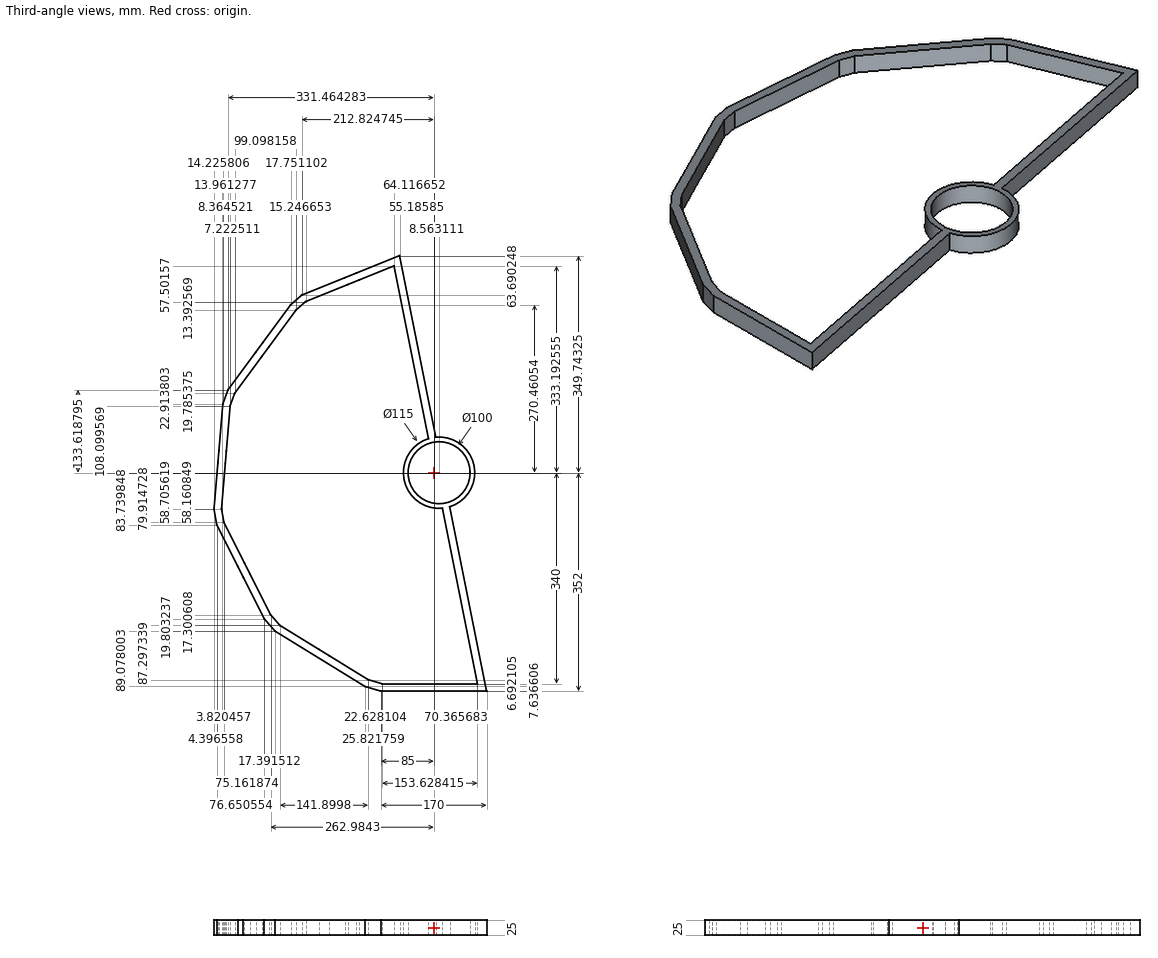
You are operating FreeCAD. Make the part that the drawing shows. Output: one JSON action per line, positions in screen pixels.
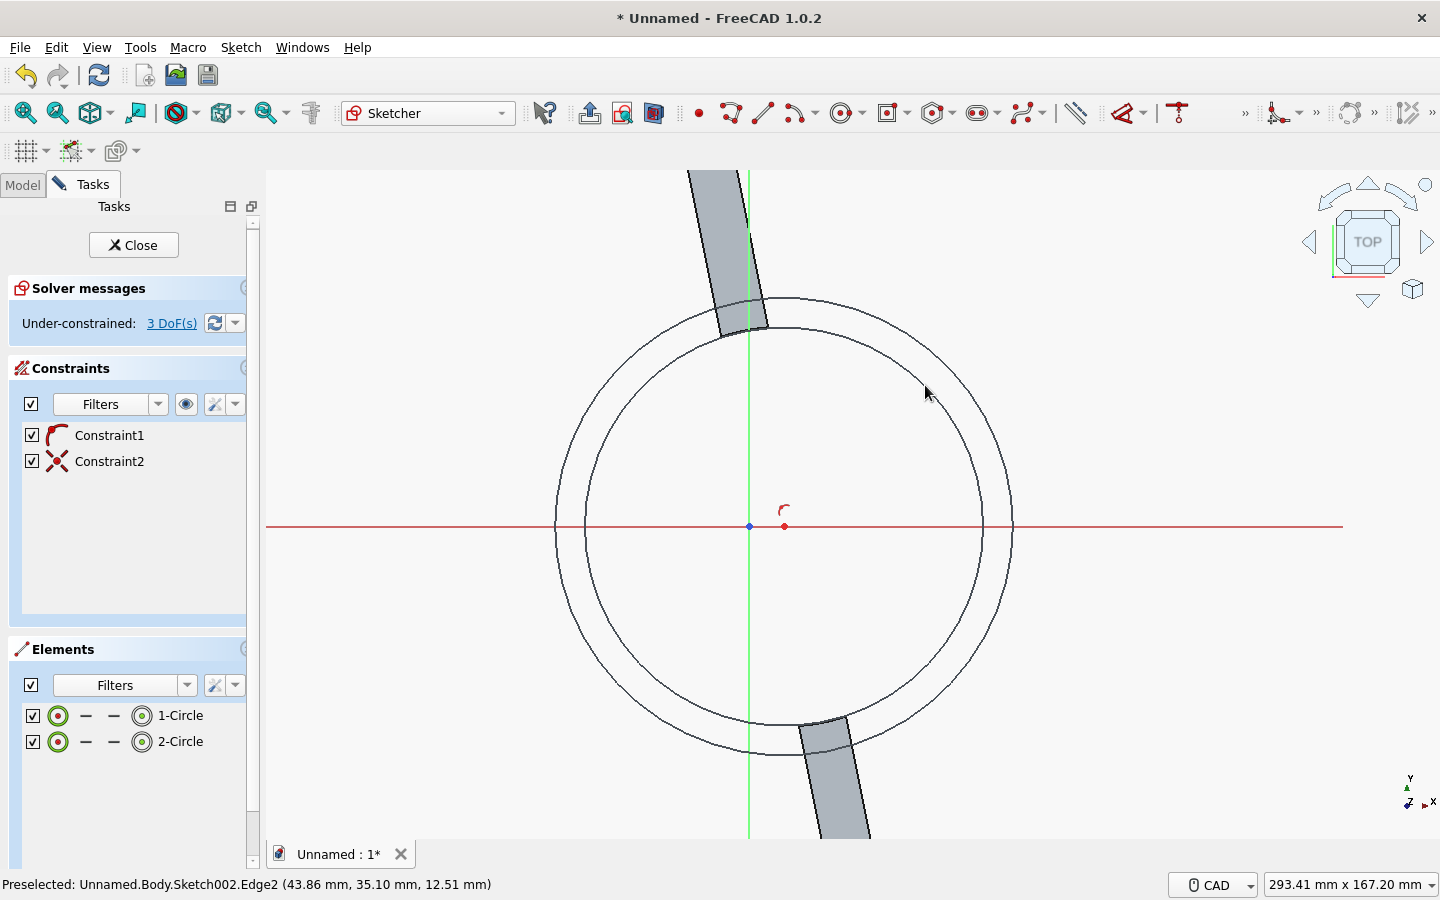
{"action": "left_click", "coordinate": [1122, 114]}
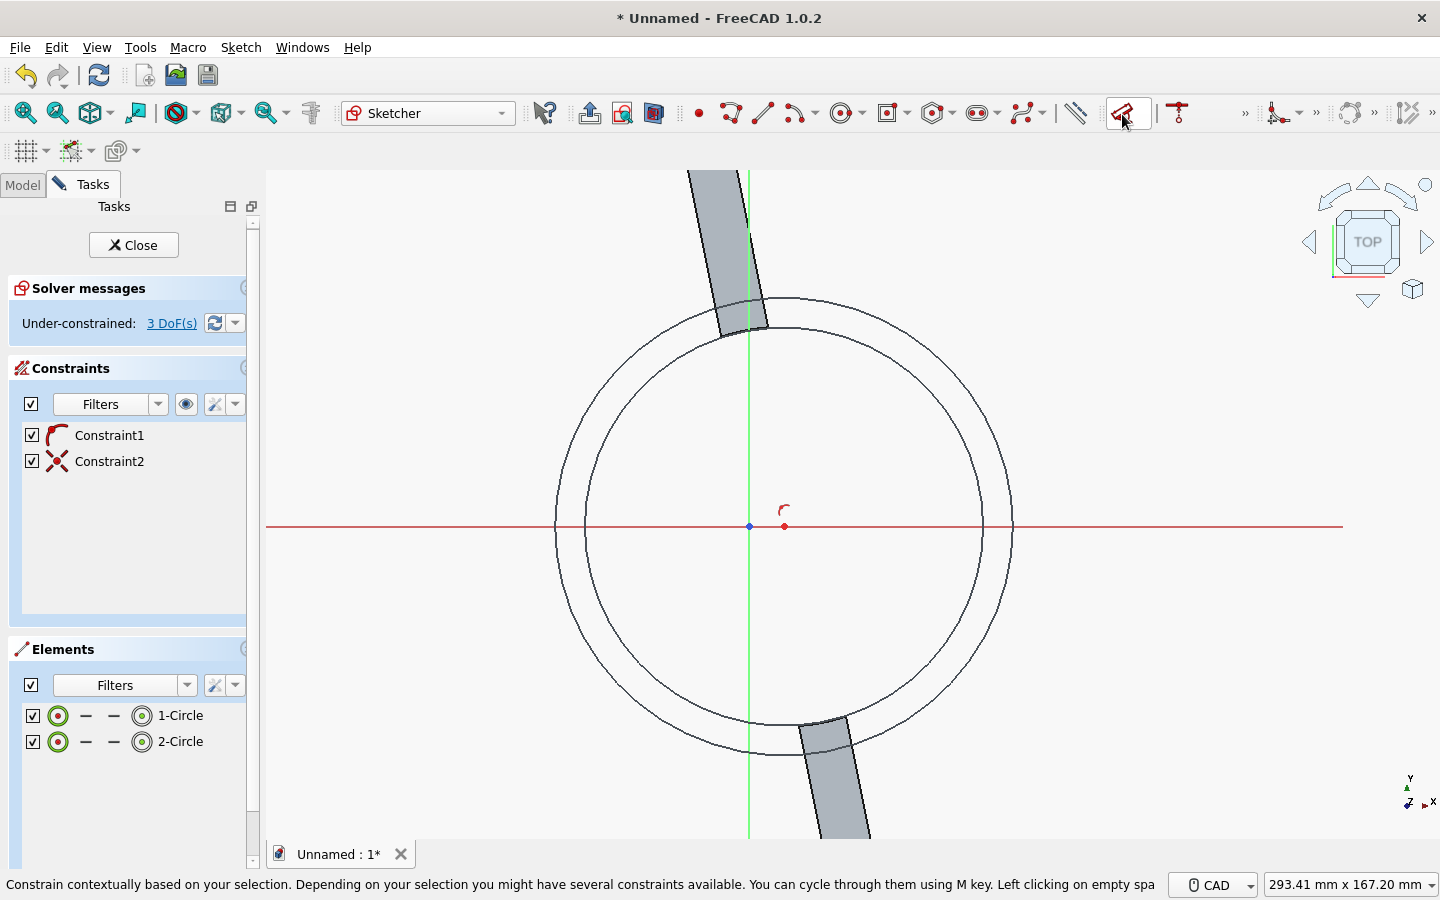
{"action": "left_click", "coordinate": [945, 364]}
{"action": "left_click", "coordinate": [968, 341]}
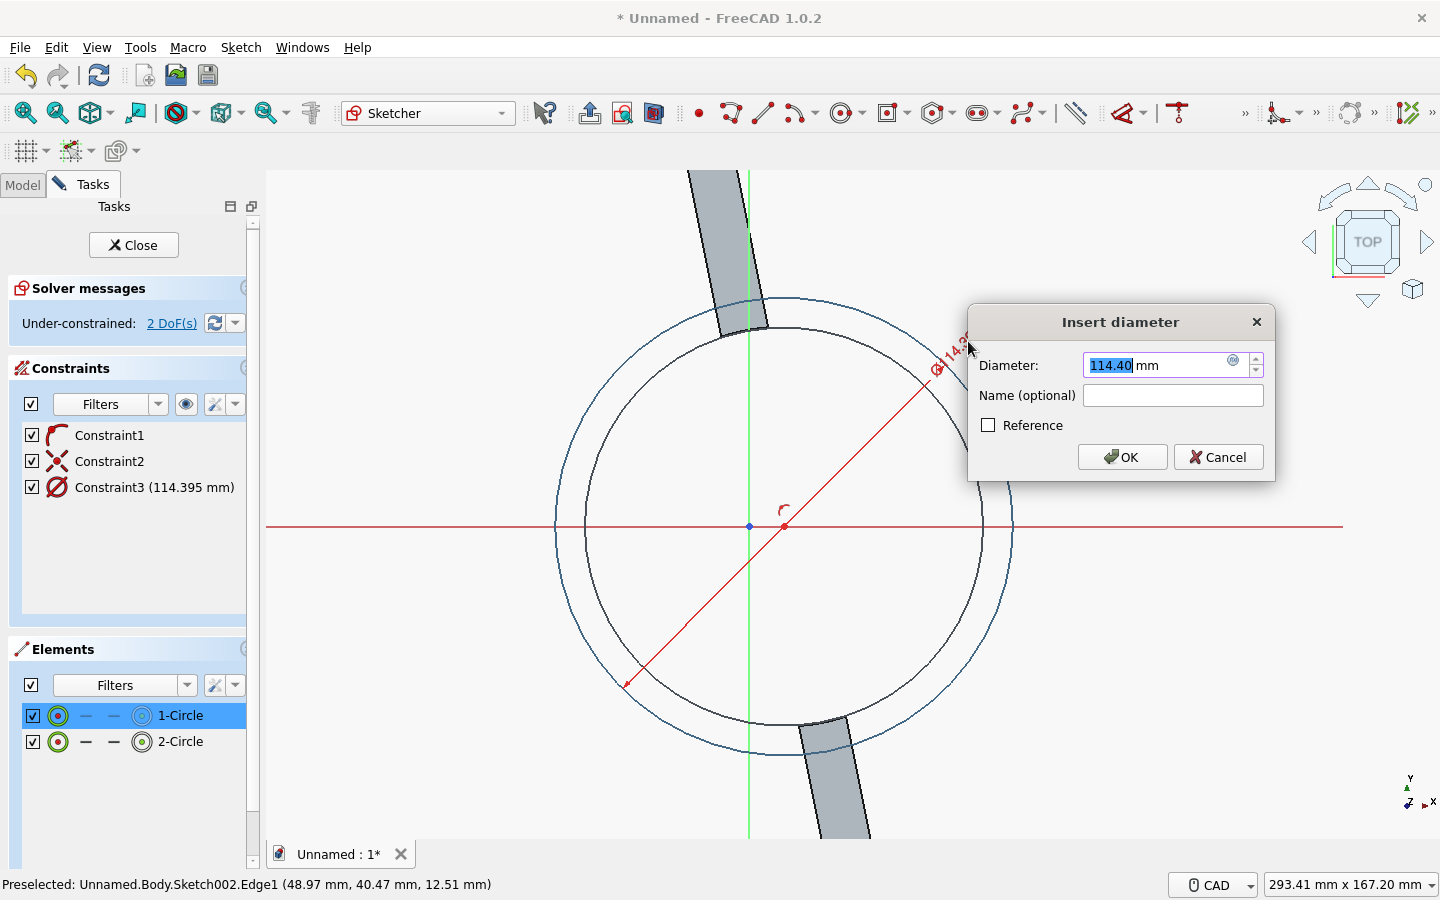
{"action": "type", "text": "115"}
{"action": "key", "text": "Return"}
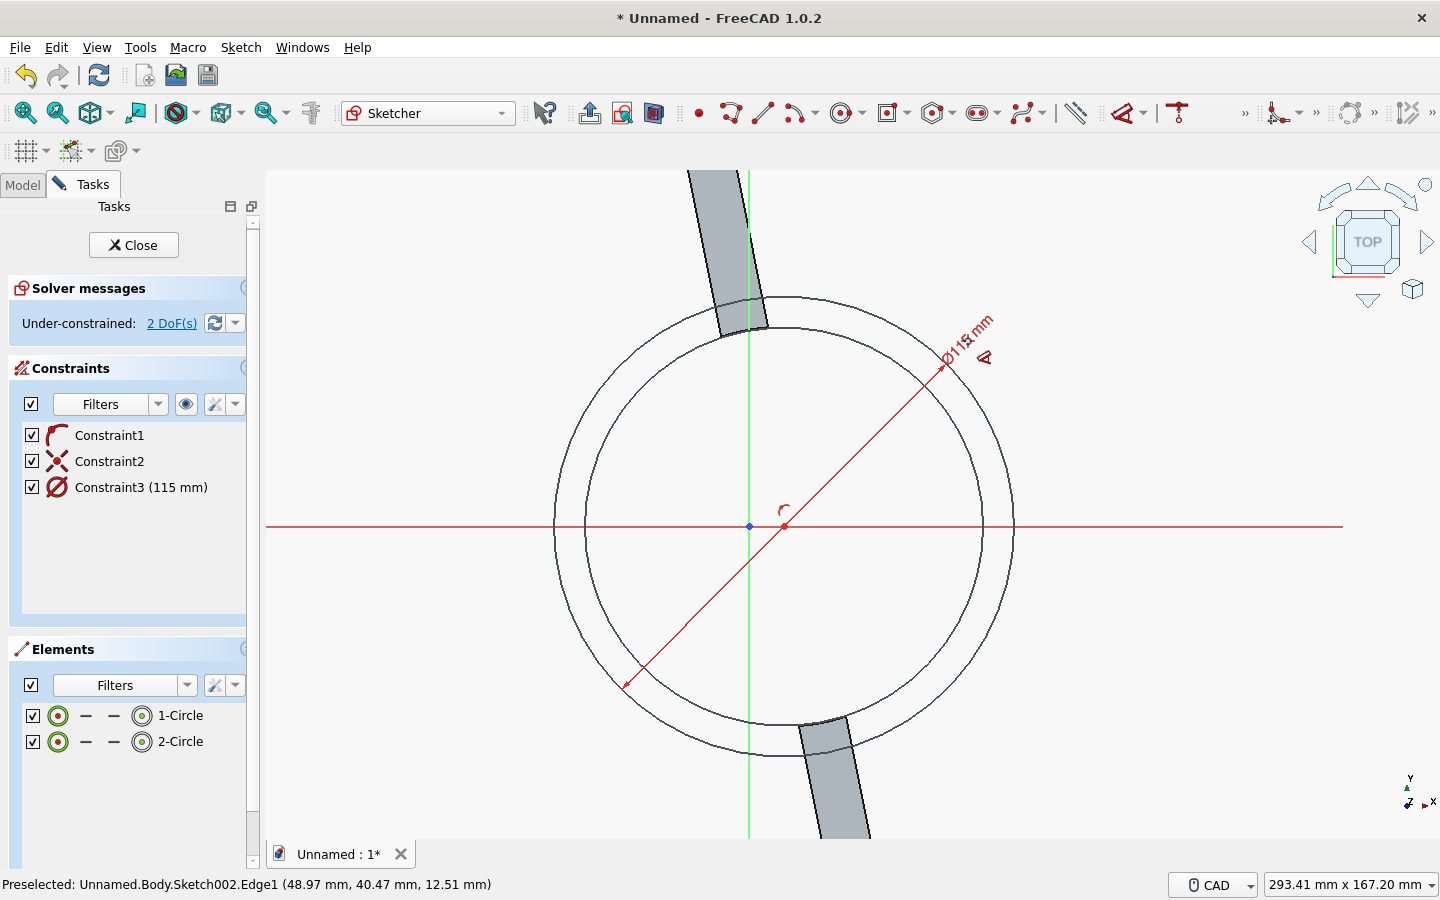
{"action": "left_click", "coordinate": [924, 385]}
{"action": "left_click", "coordinate": [1027, 454]}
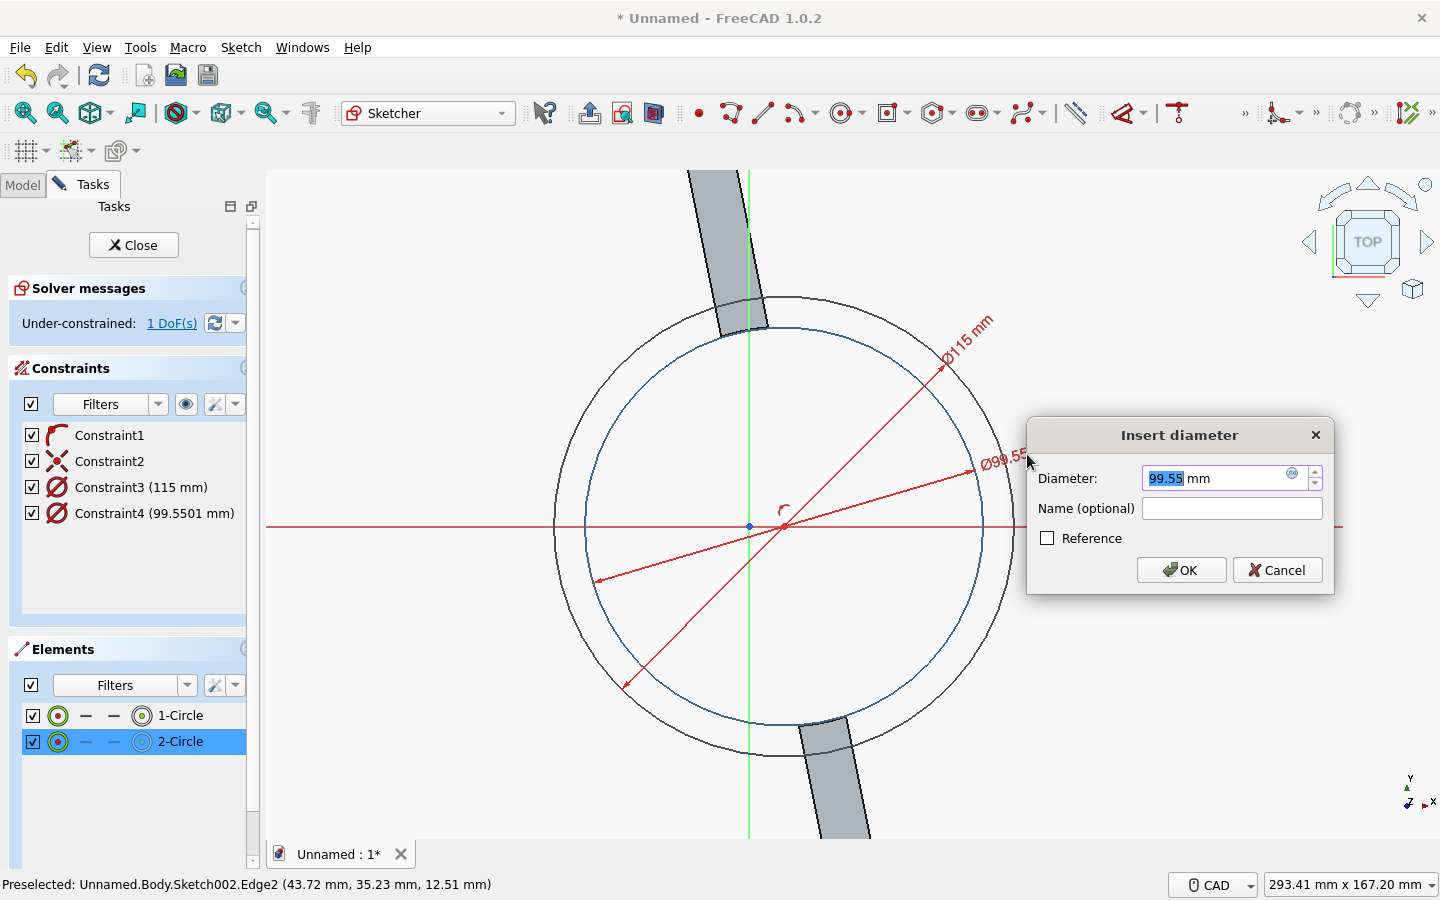
{"action": "type", "text": "100"}
{"action": "key", "text": "Return"}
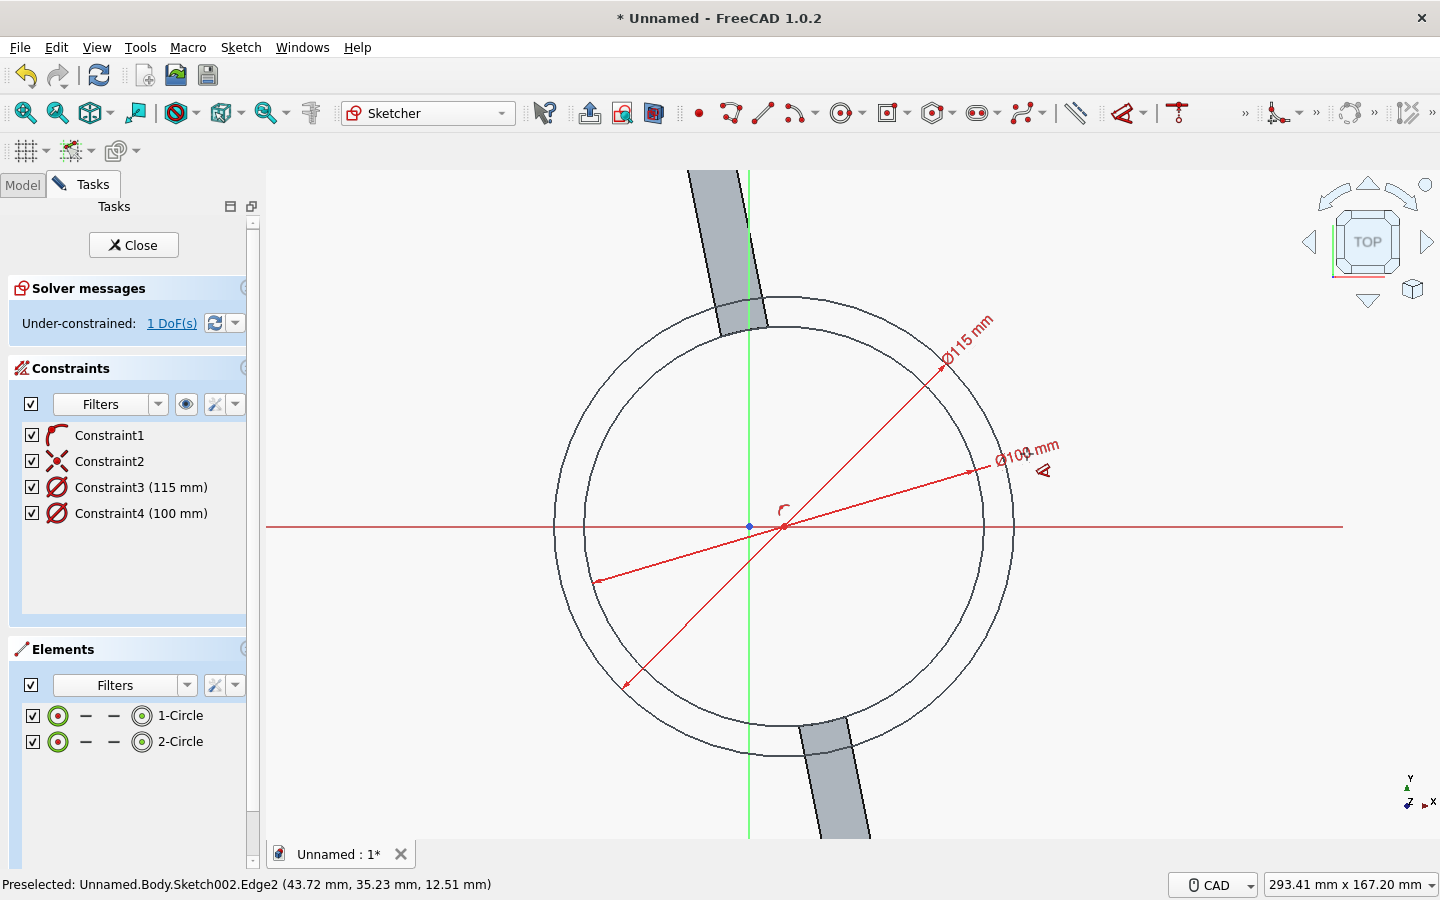
{"action": "left_click", "coordinate": [784, 527]}
{"action": "left_click", "coordinate": [767, 561]}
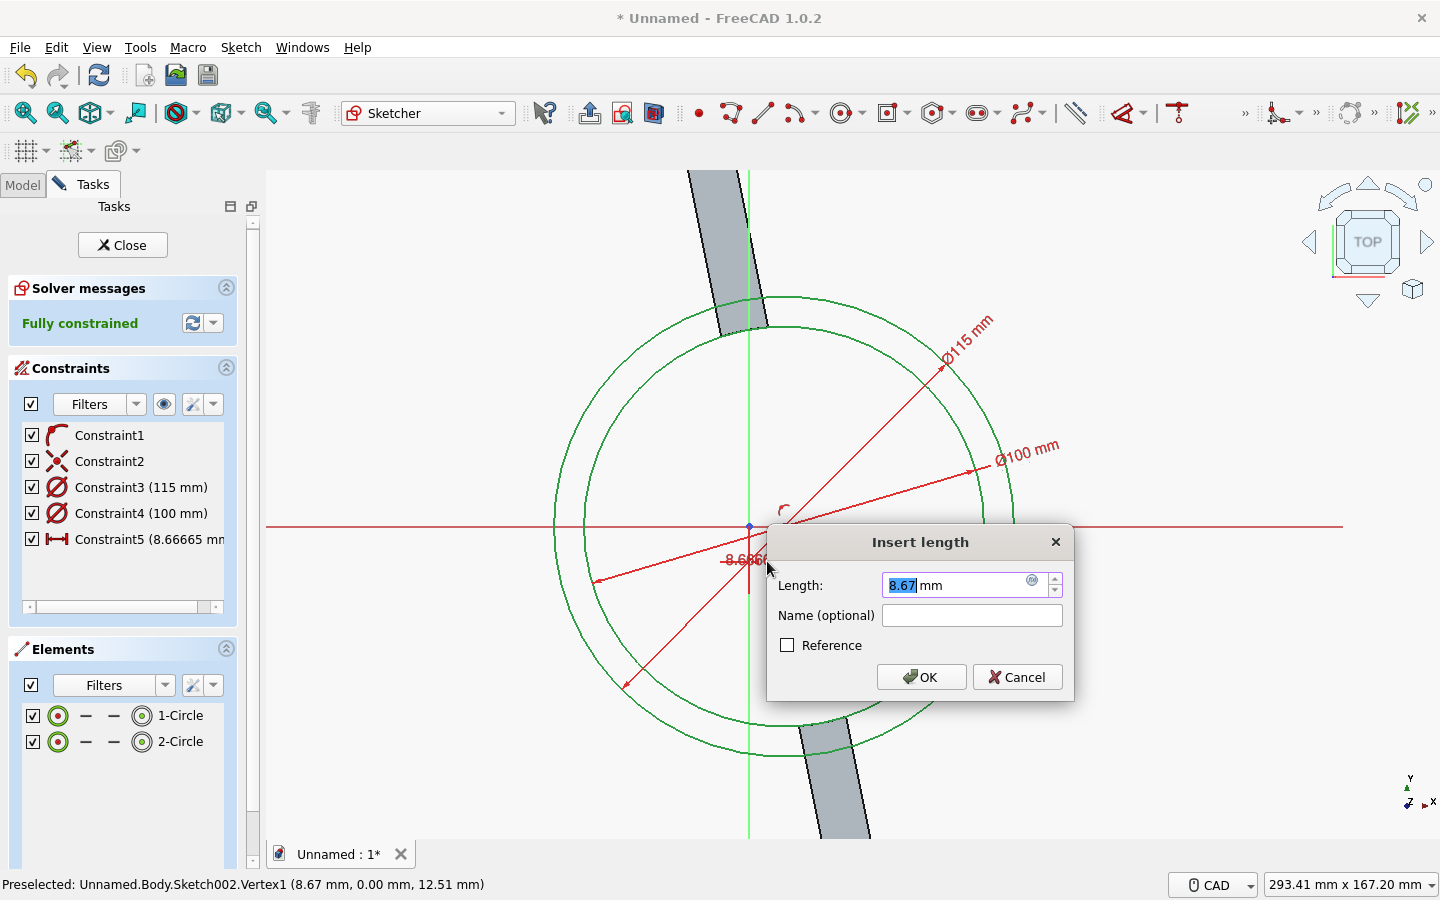
{"action": "type", "text": "8.563111"}
{"action": "key", "text": "Return"}
{"action": "key", "text": "Escape"}